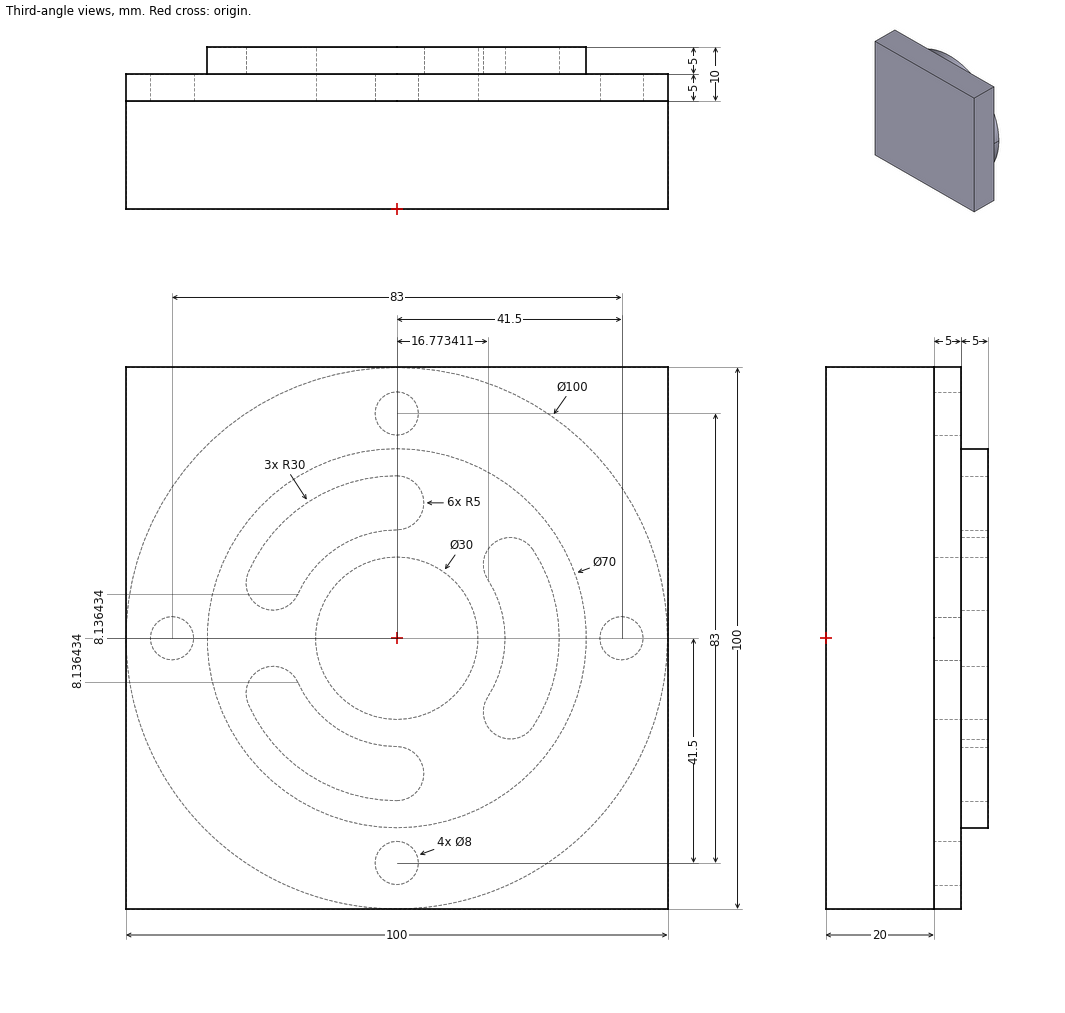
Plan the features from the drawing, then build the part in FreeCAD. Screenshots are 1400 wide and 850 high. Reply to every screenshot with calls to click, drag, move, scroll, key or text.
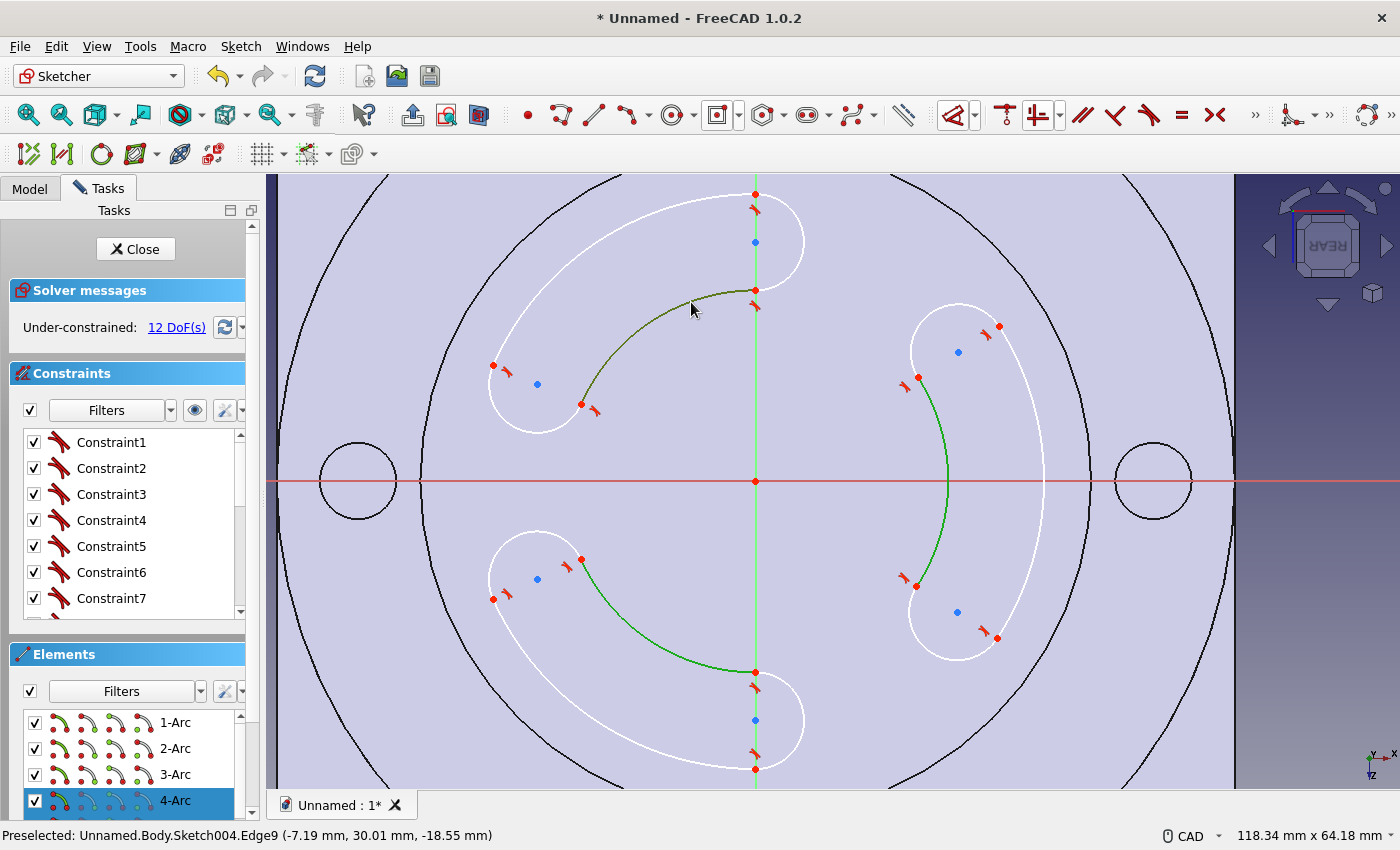
click(1182, 116)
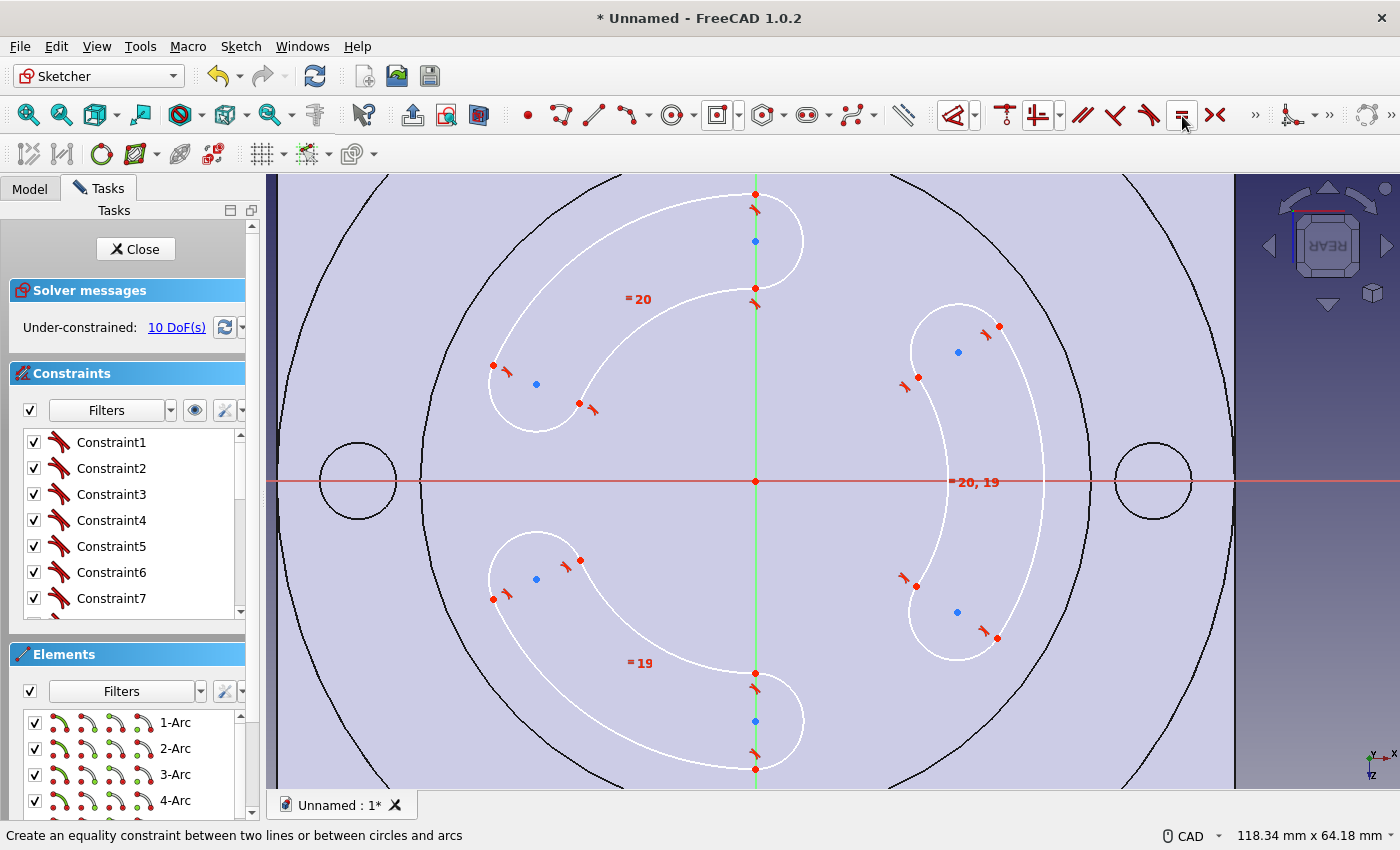
click(546, 533)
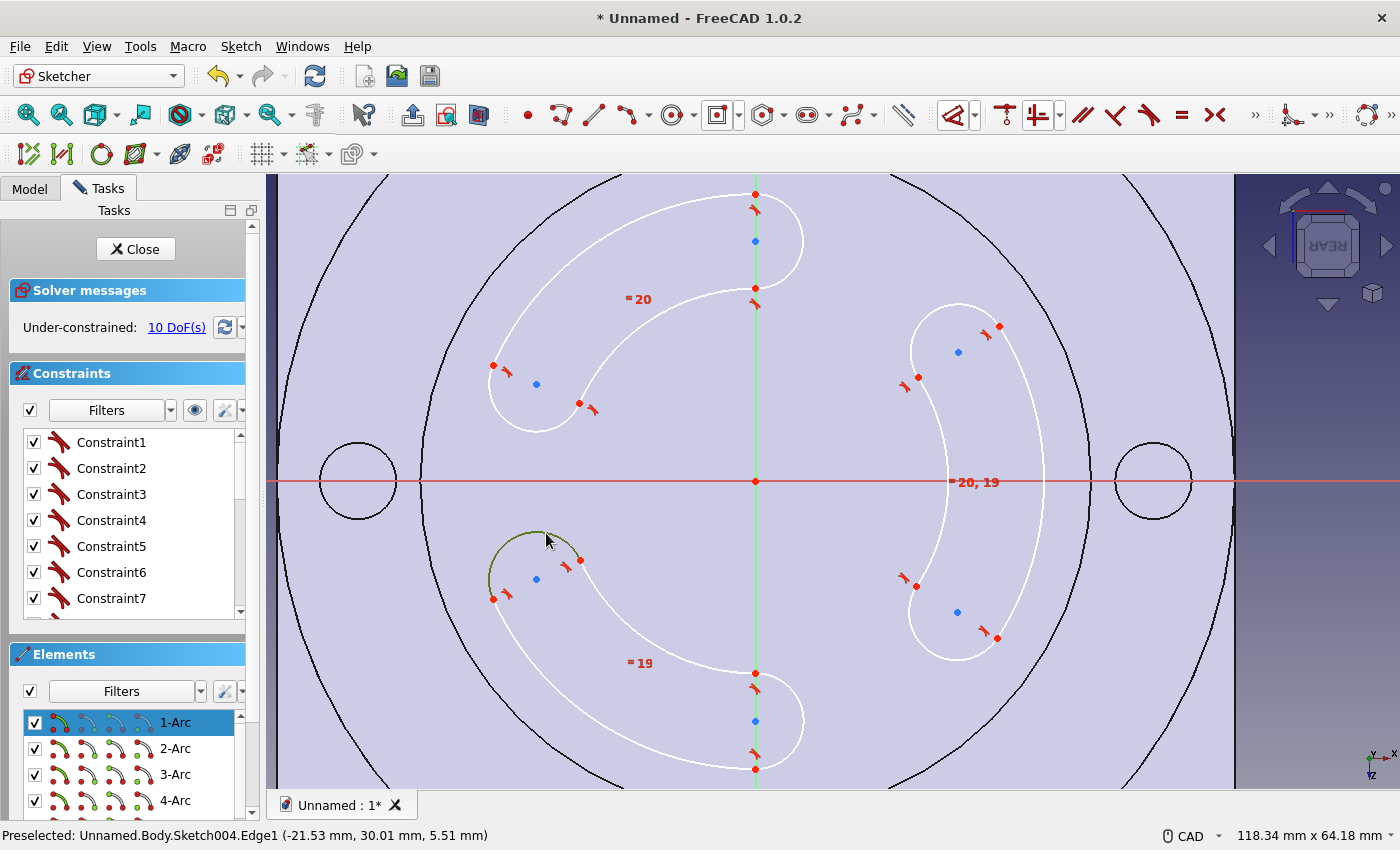
click(912, 629)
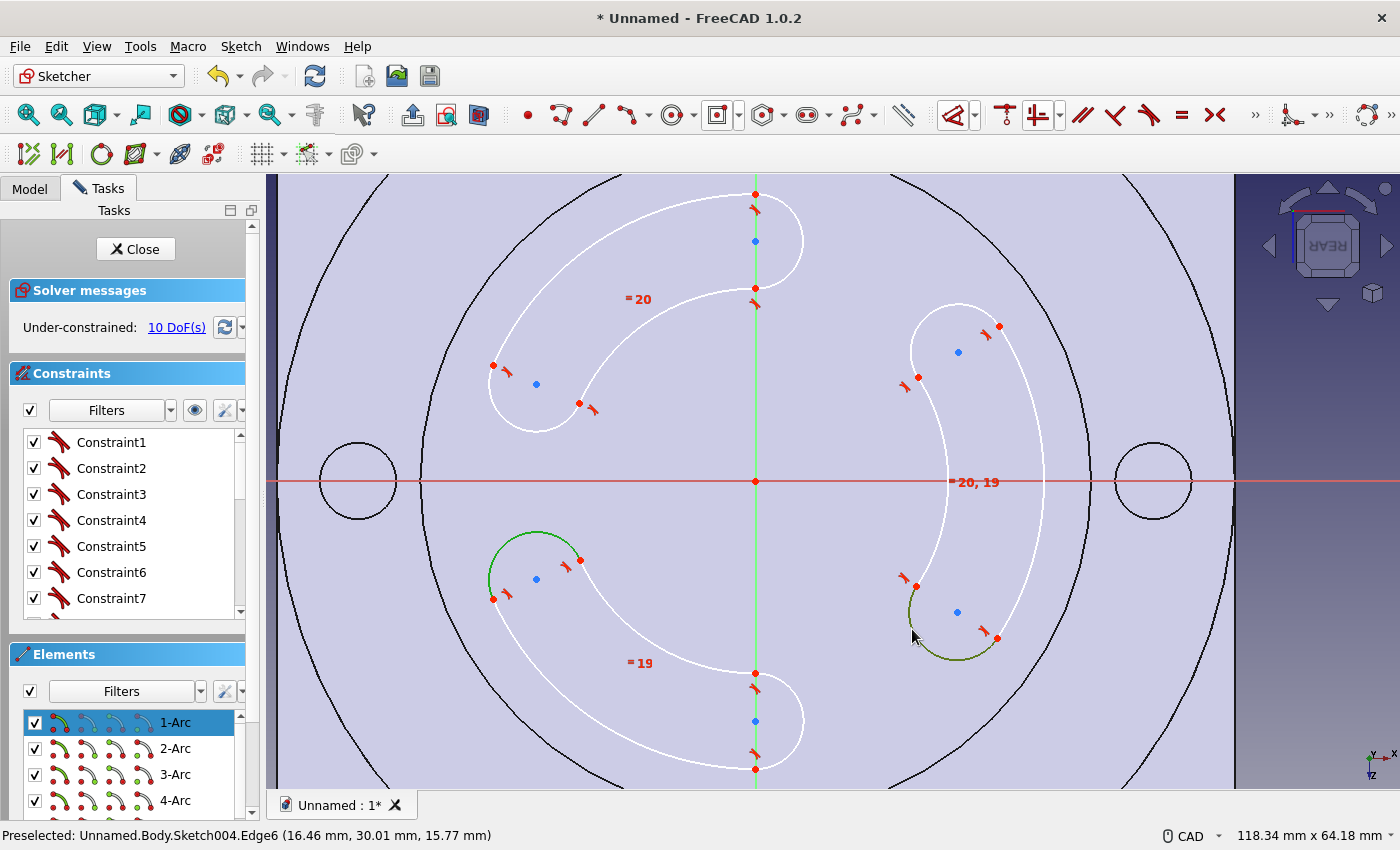
click(794, 269)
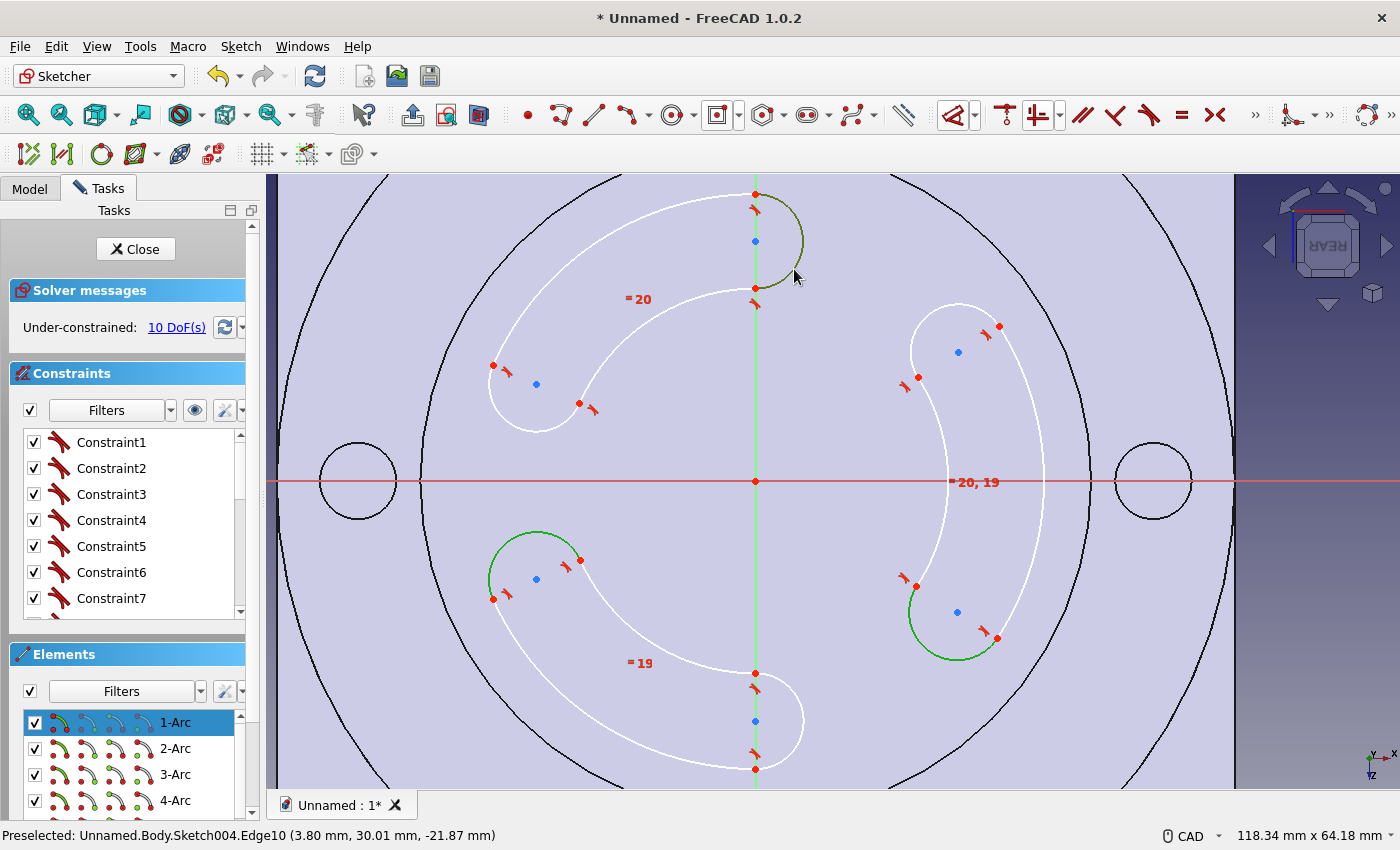
click(1182, 116)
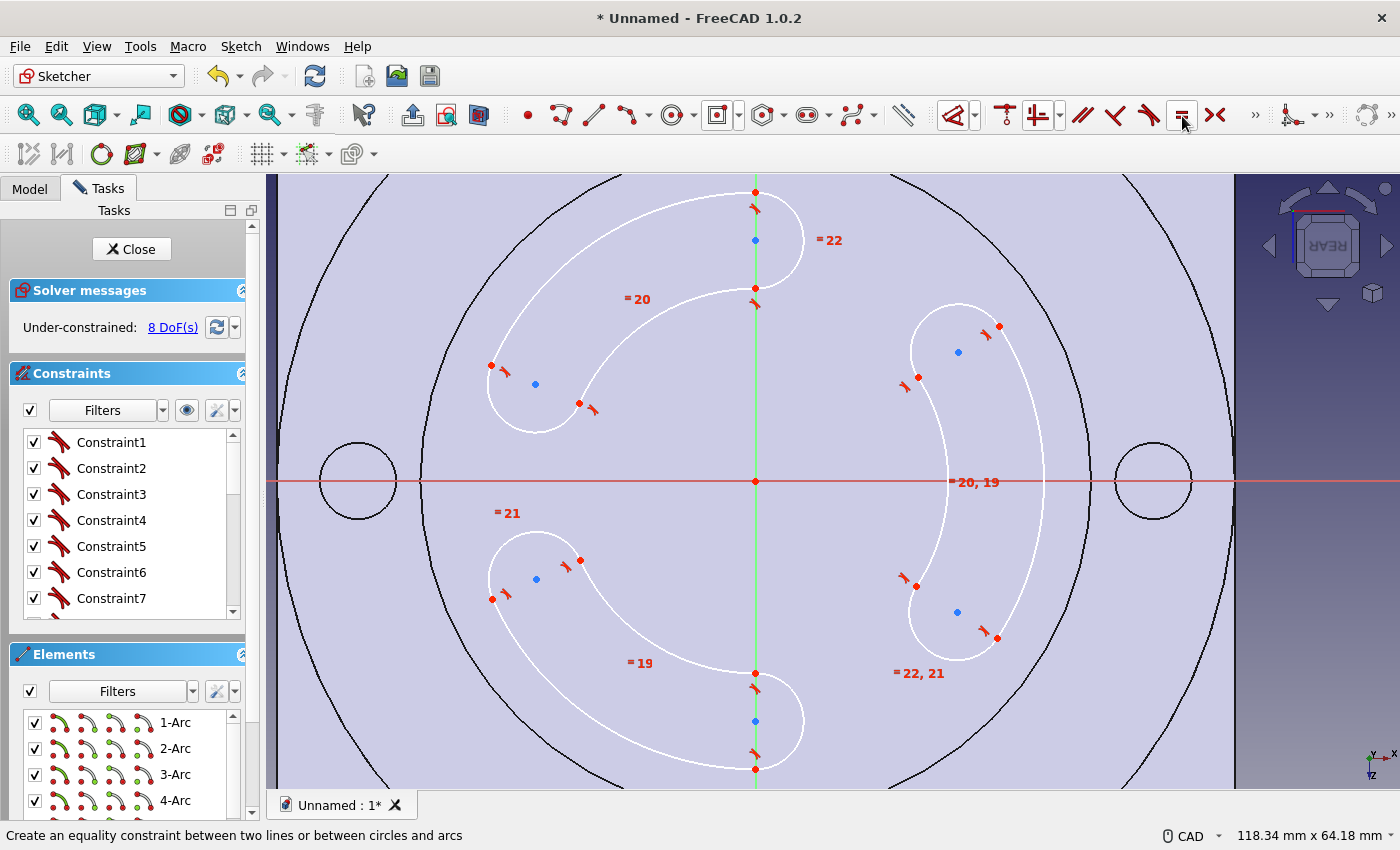
click(756, 721)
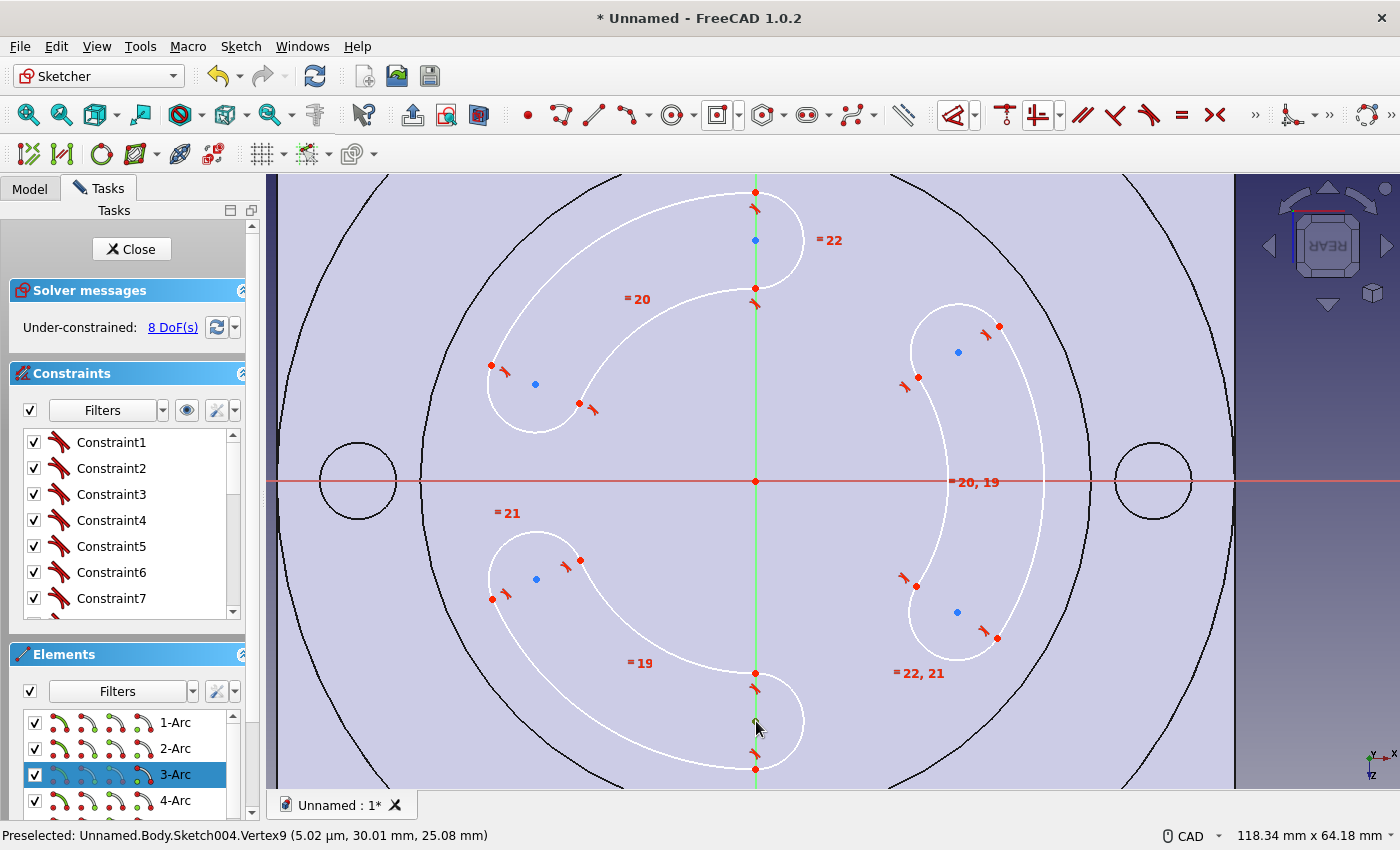
click(756, 641)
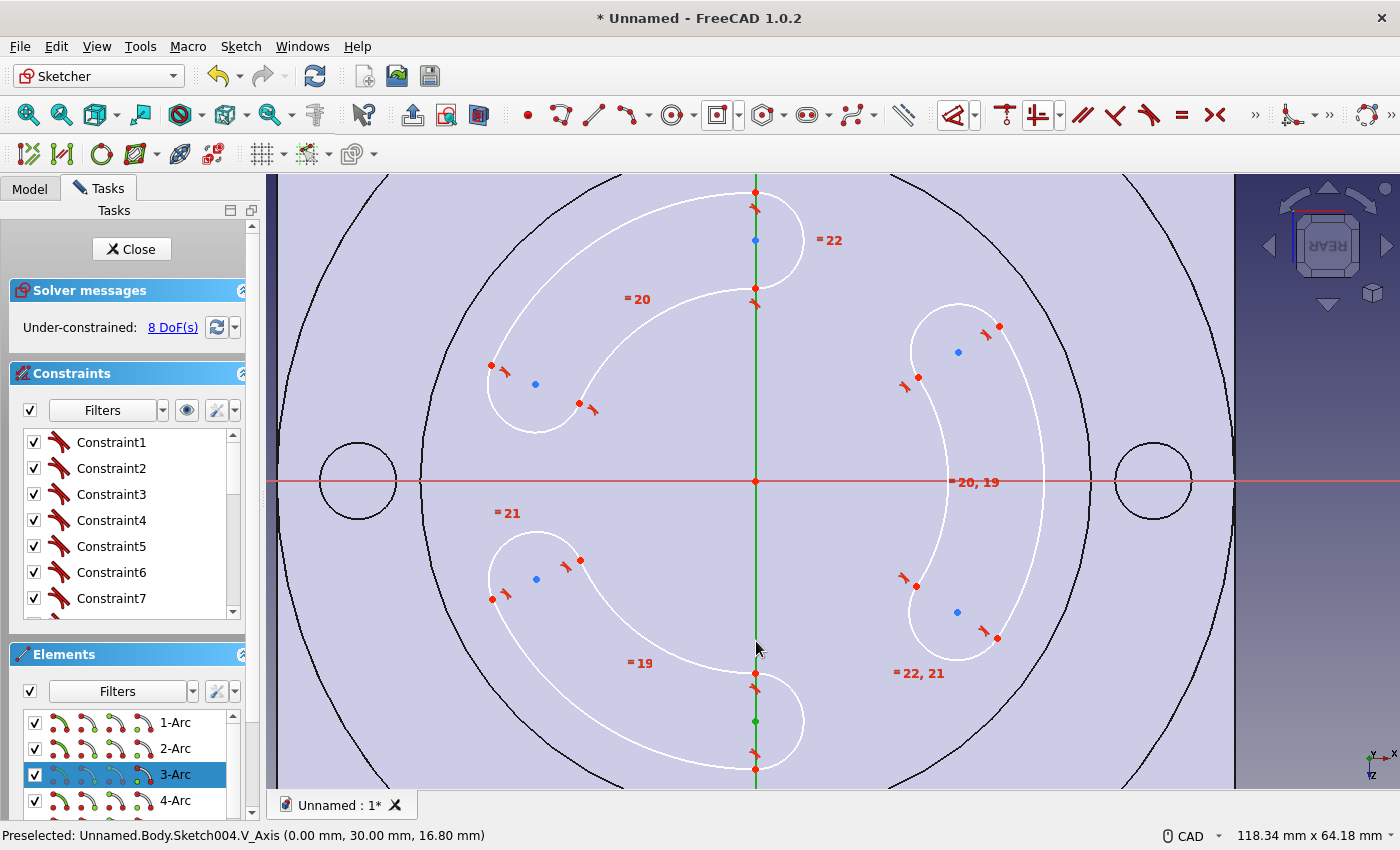
click(1005, 116)